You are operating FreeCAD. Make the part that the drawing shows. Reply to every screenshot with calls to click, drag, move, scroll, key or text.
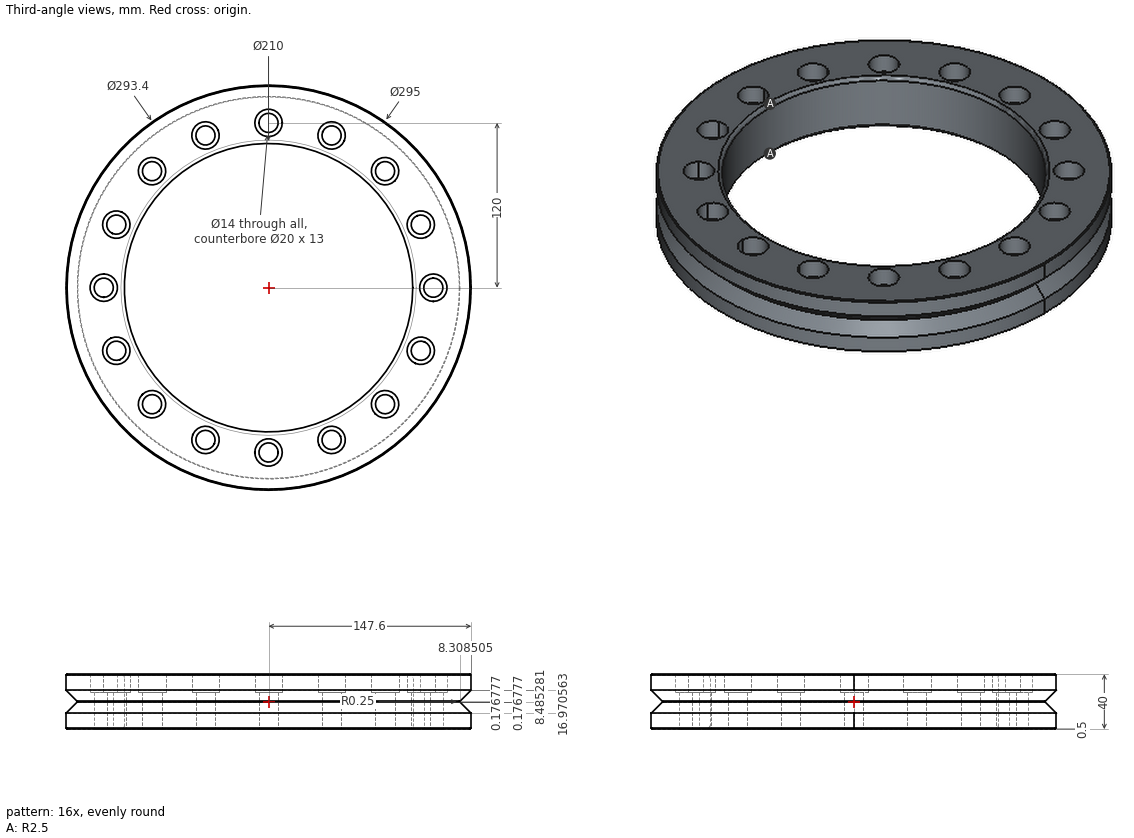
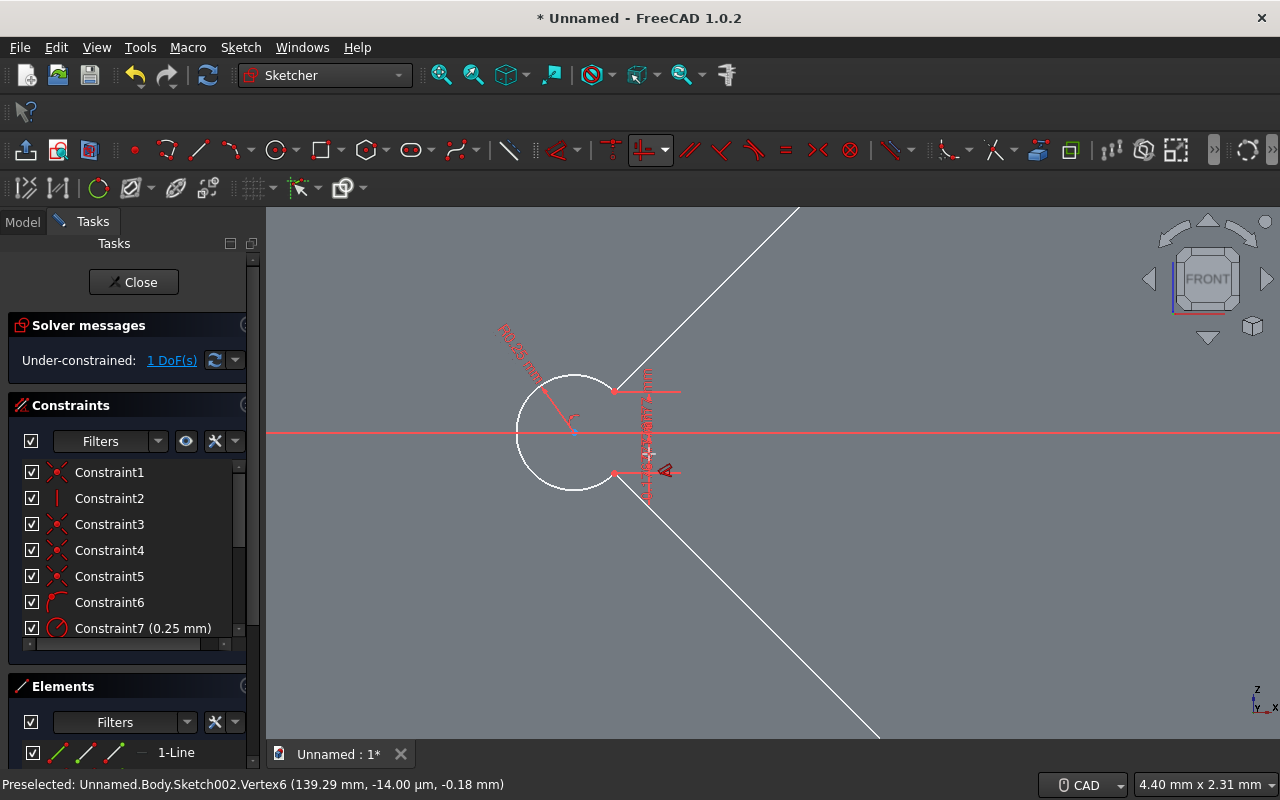
scroll(623, 477, down, 12)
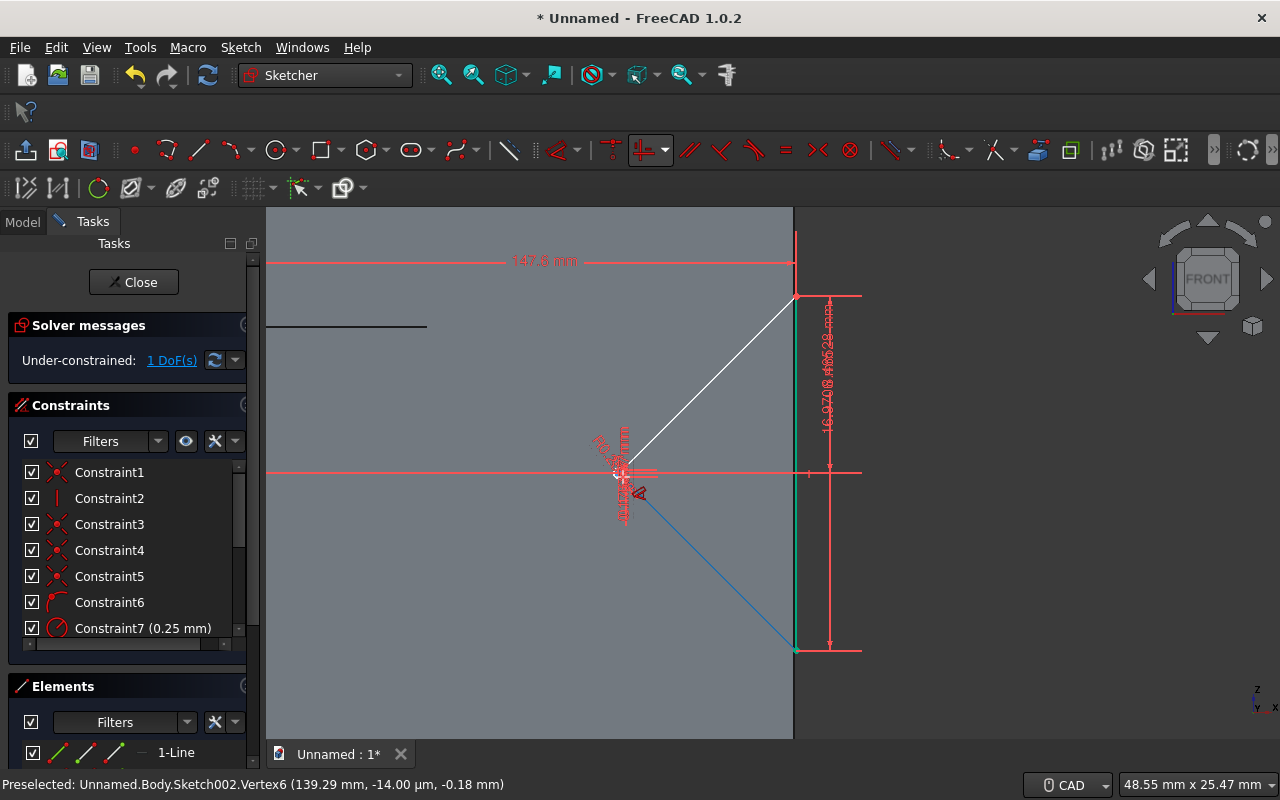
click(675, 418)
click(709, 262)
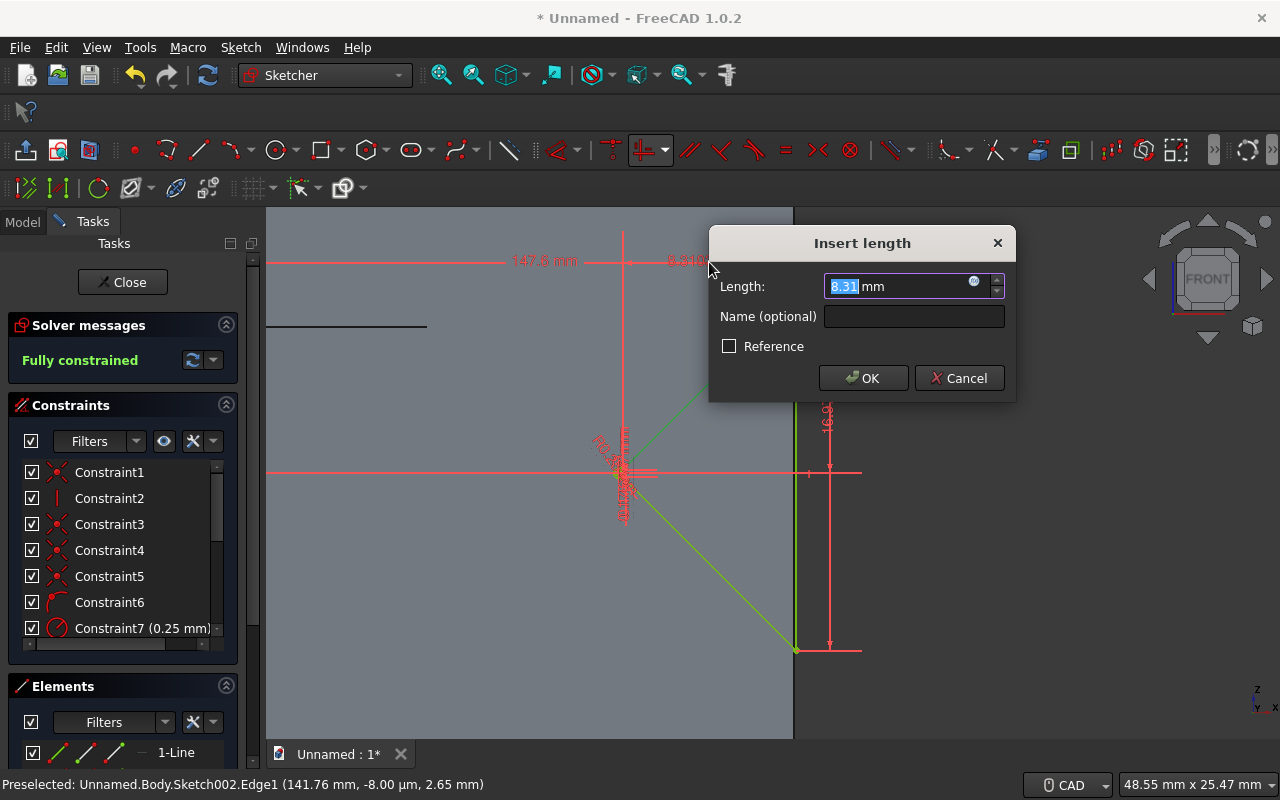
text(8.308505)
key(Return)
key(Escape)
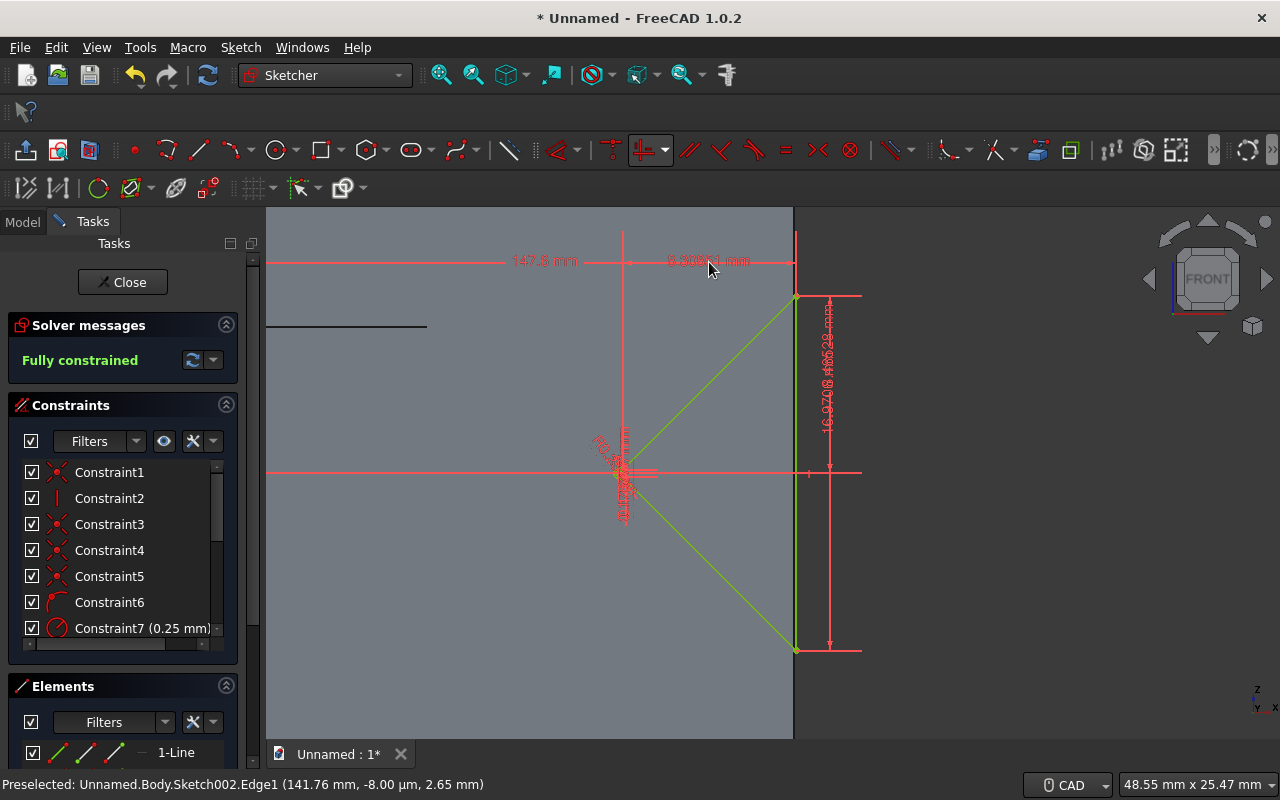
click(123, 282)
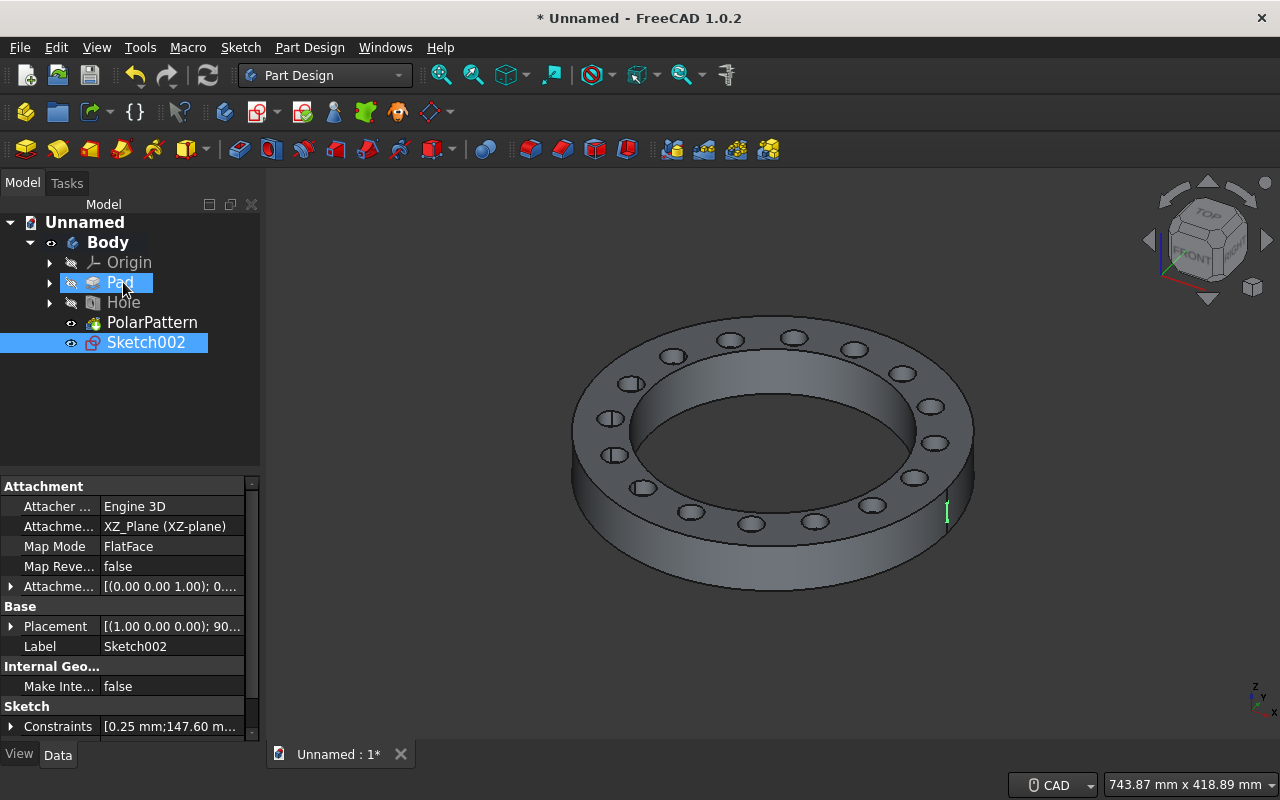
click(304, 150)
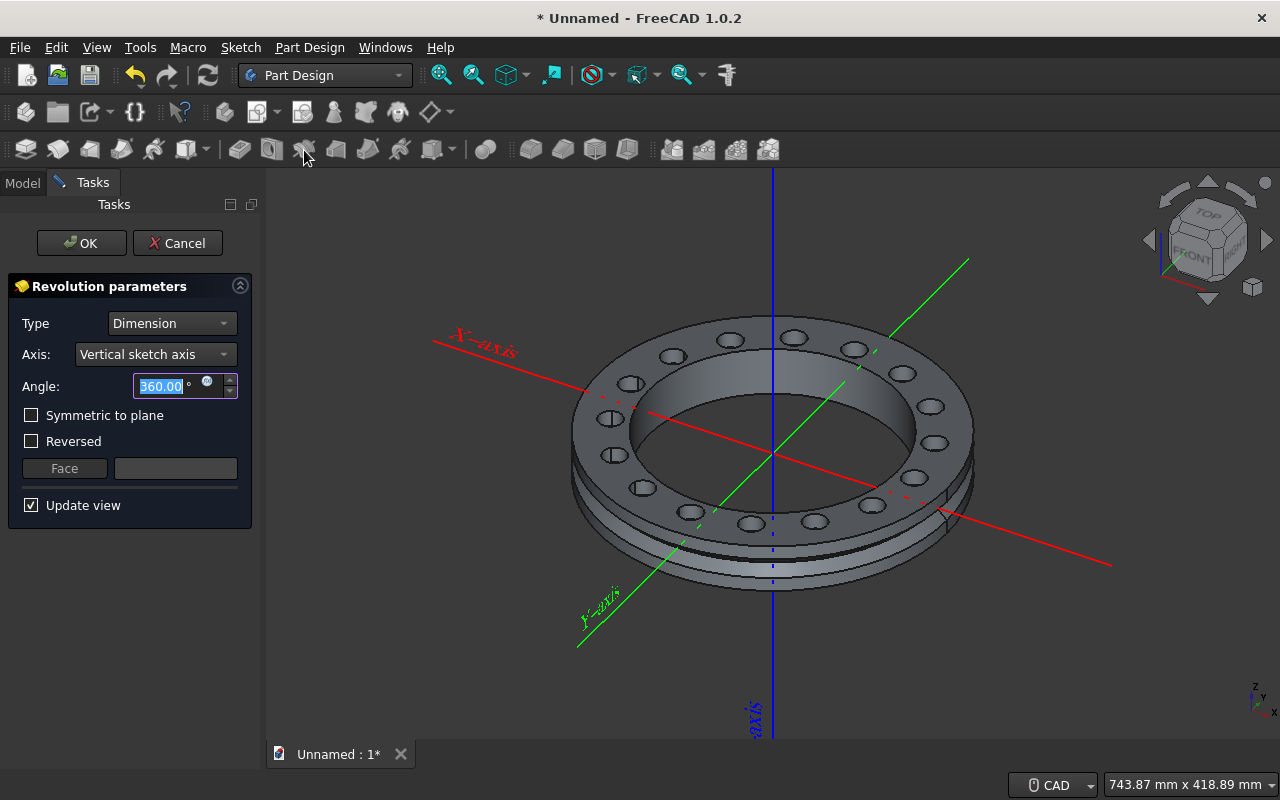
click(82, 243)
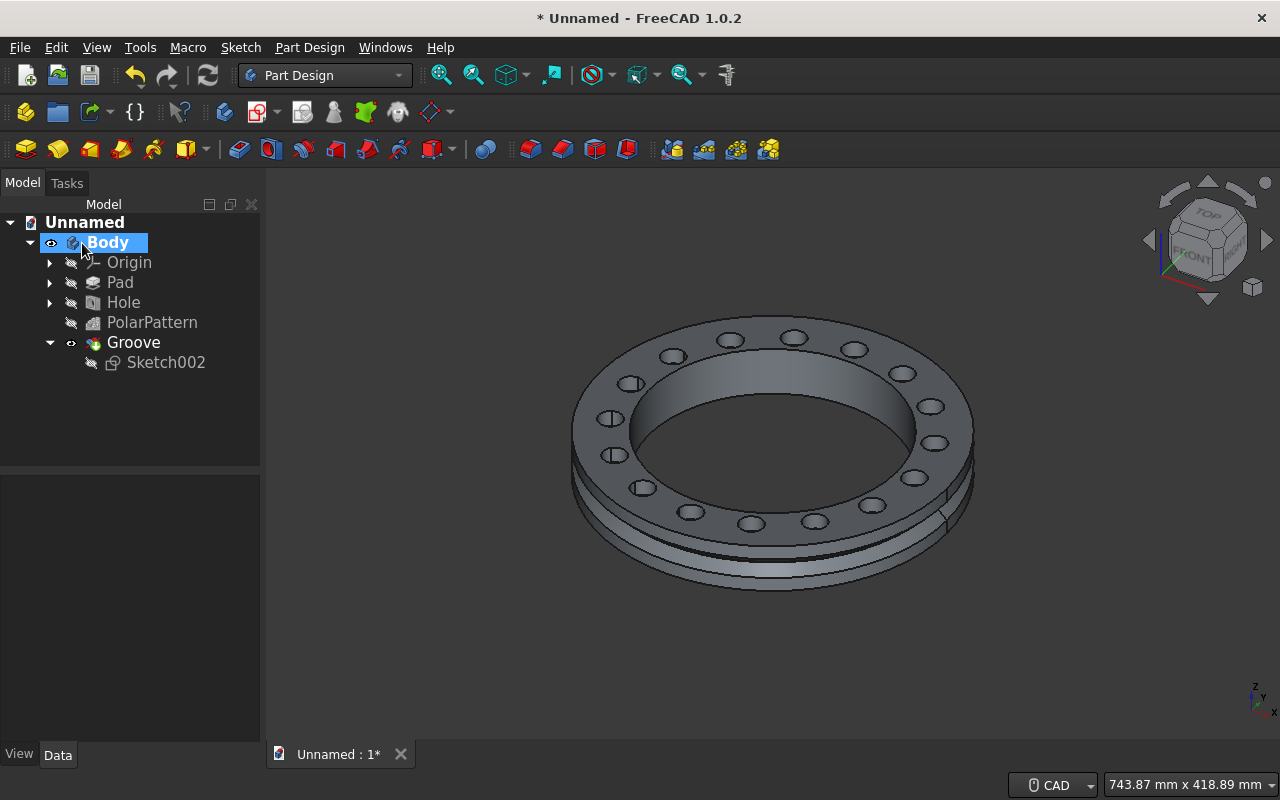
click(50, 263)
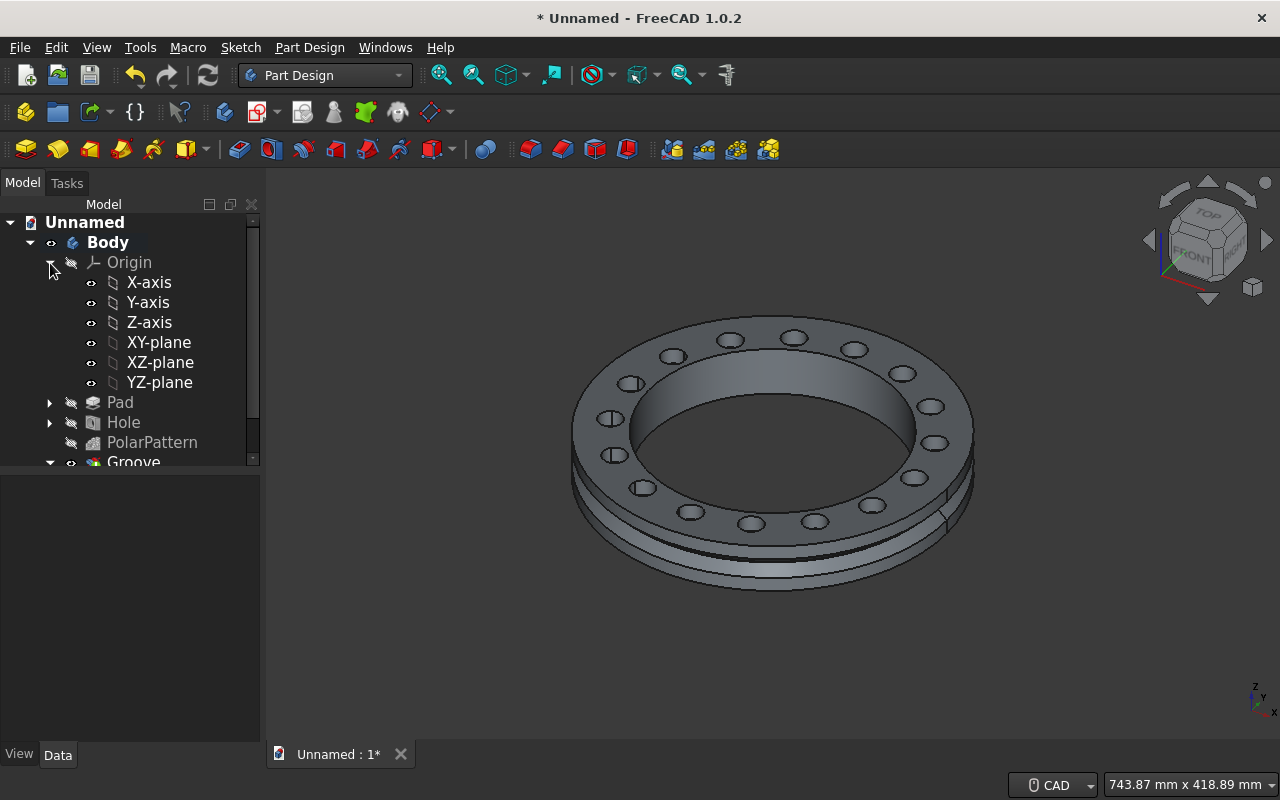
click(136, 343)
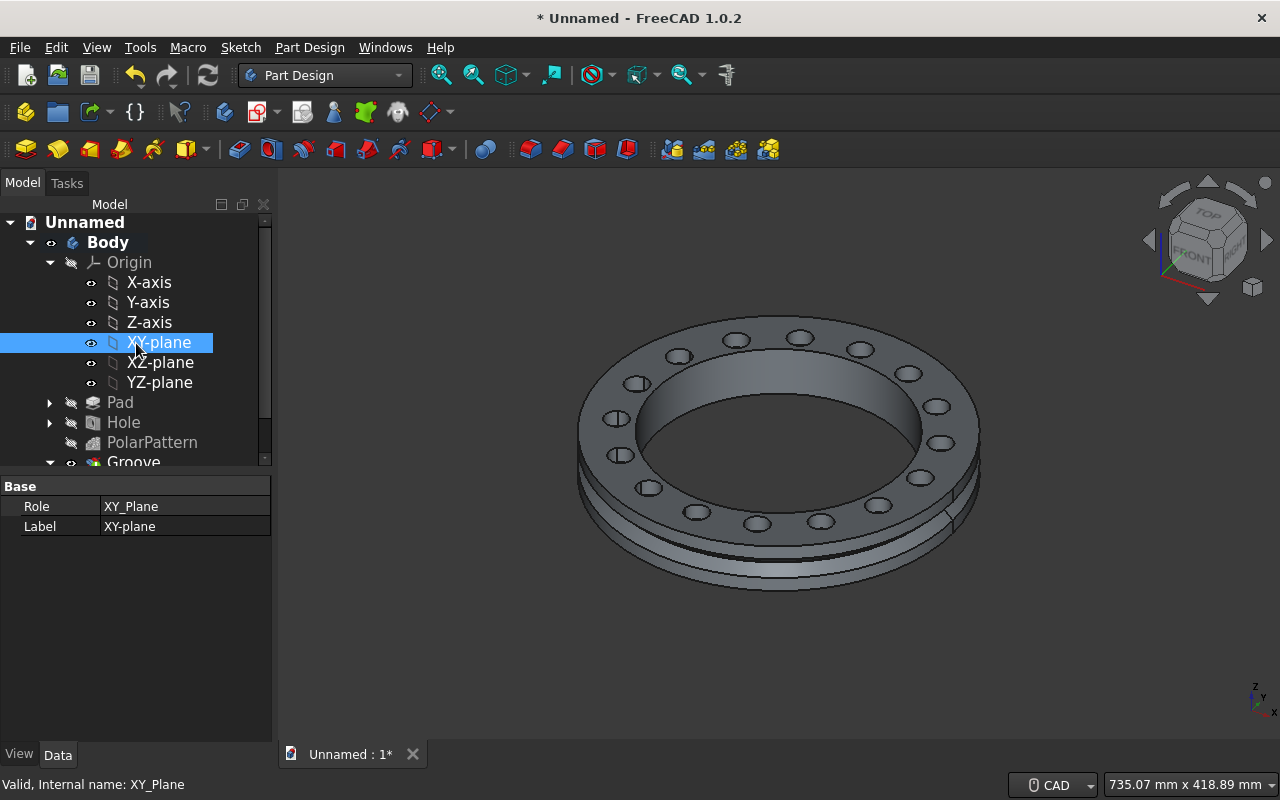
click(430, 112)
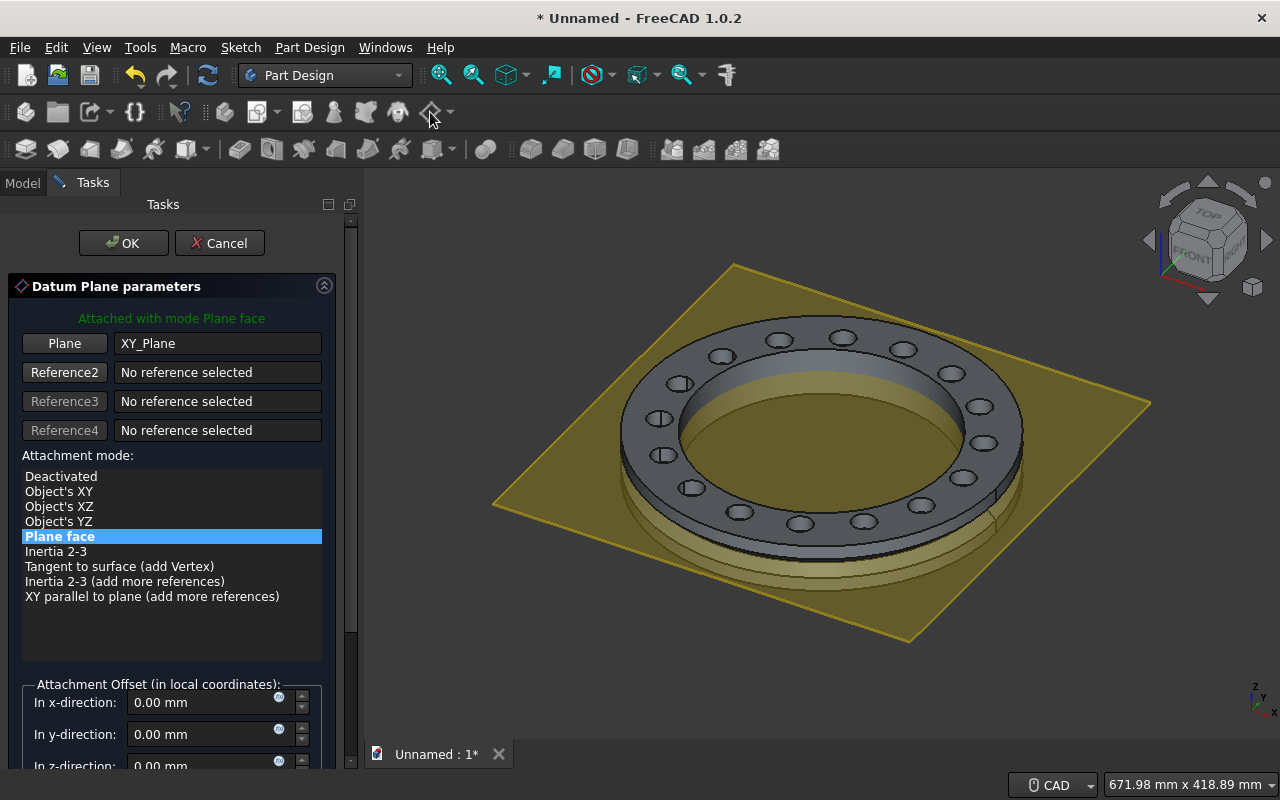
scroll(351, 491, down, 2)